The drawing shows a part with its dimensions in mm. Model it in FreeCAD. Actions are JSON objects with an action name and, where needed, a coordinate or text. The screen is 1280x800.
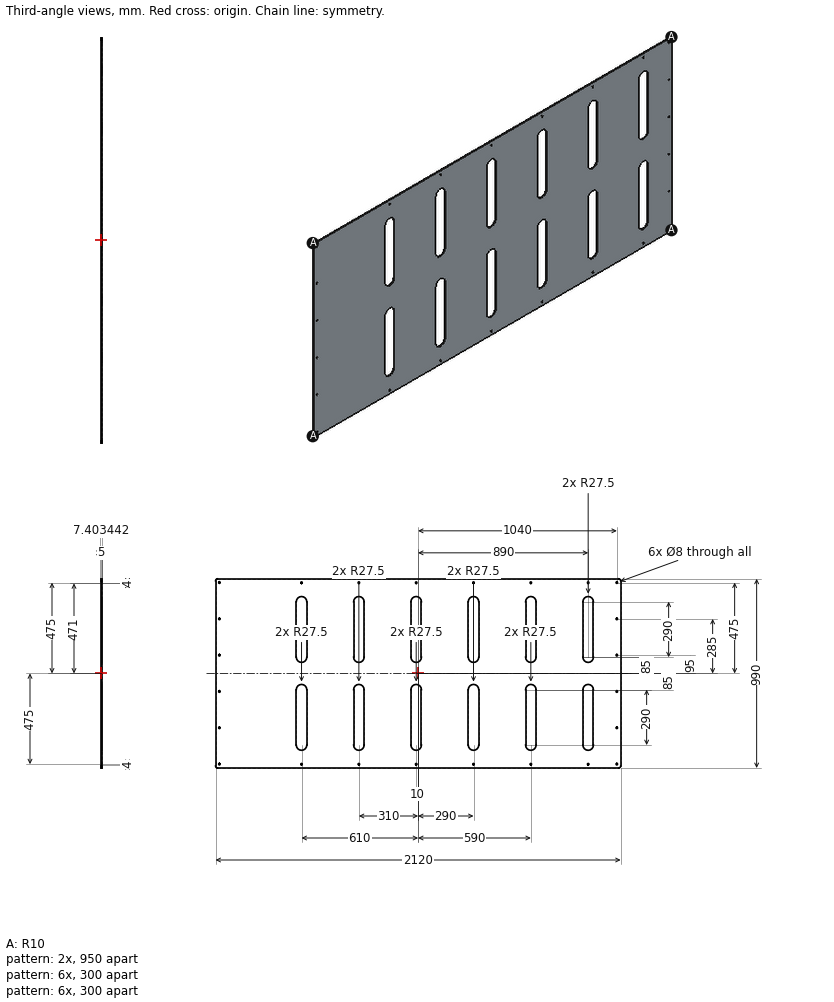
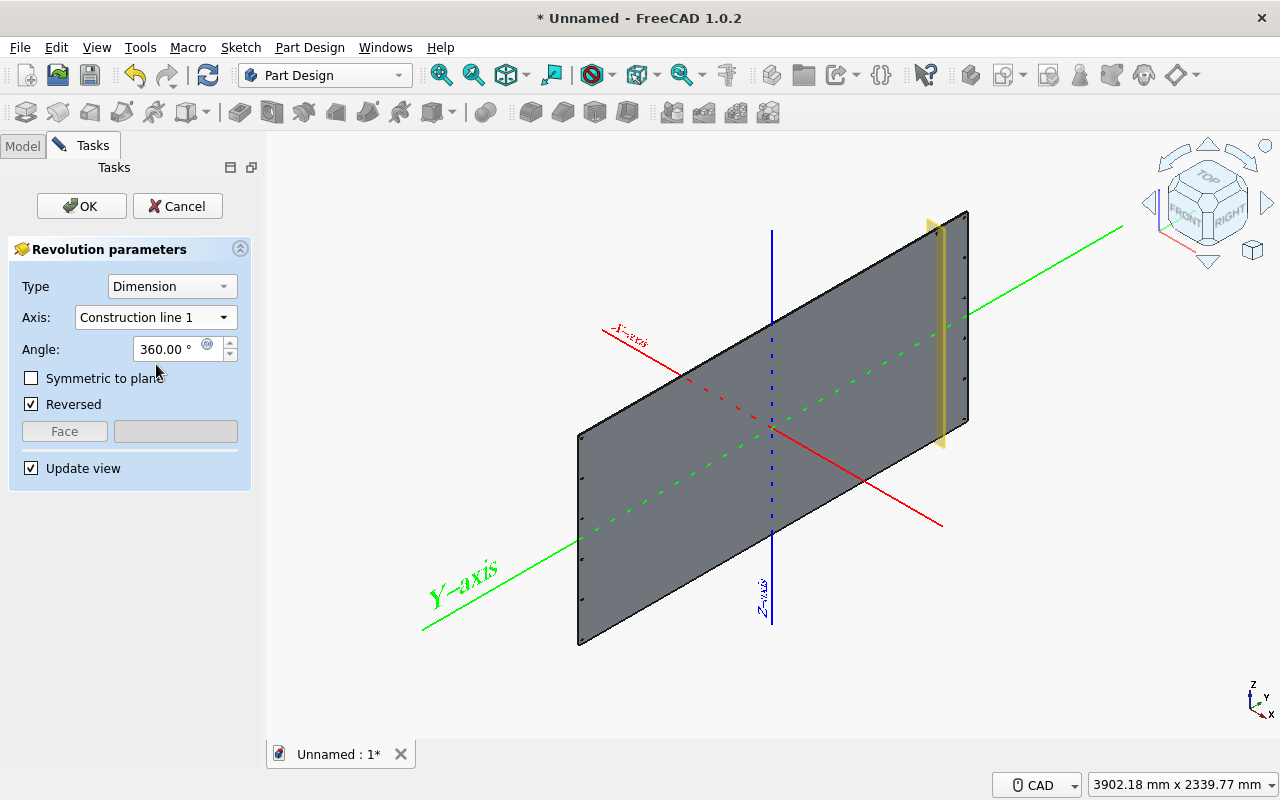
{"action": "left_click", "coordinate": [82, 206]}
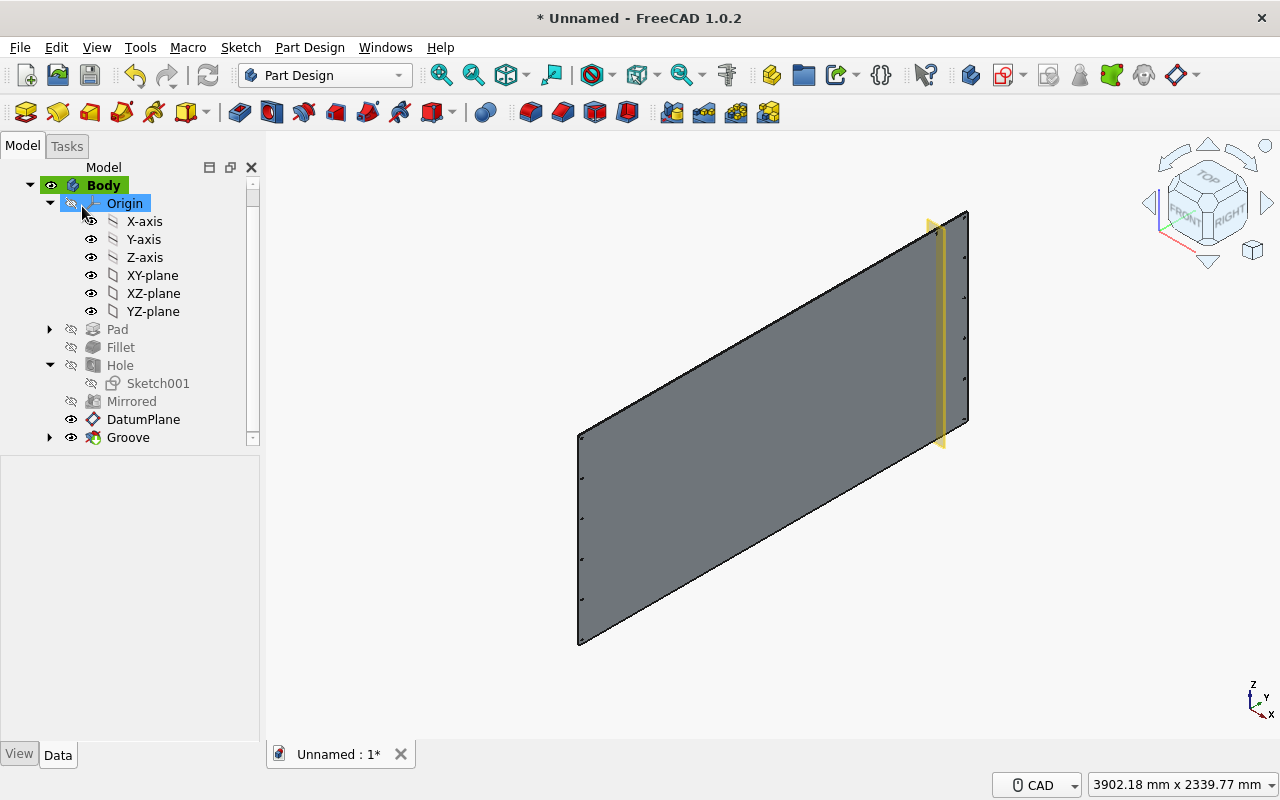
{"action": "left_click", "coordinate": [116, 419]}
{"action": "key", "text": "space"}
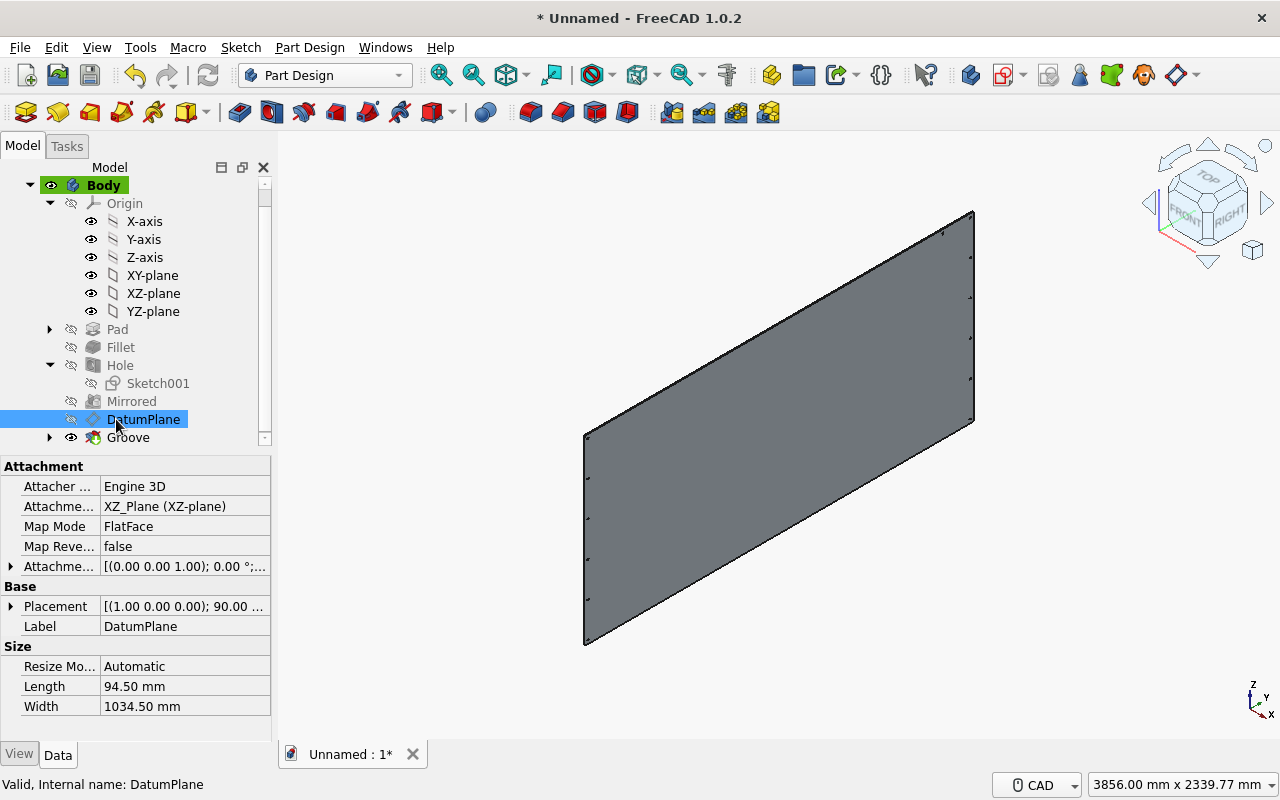
{"action": "left_click", "coordinate": [116, 437]}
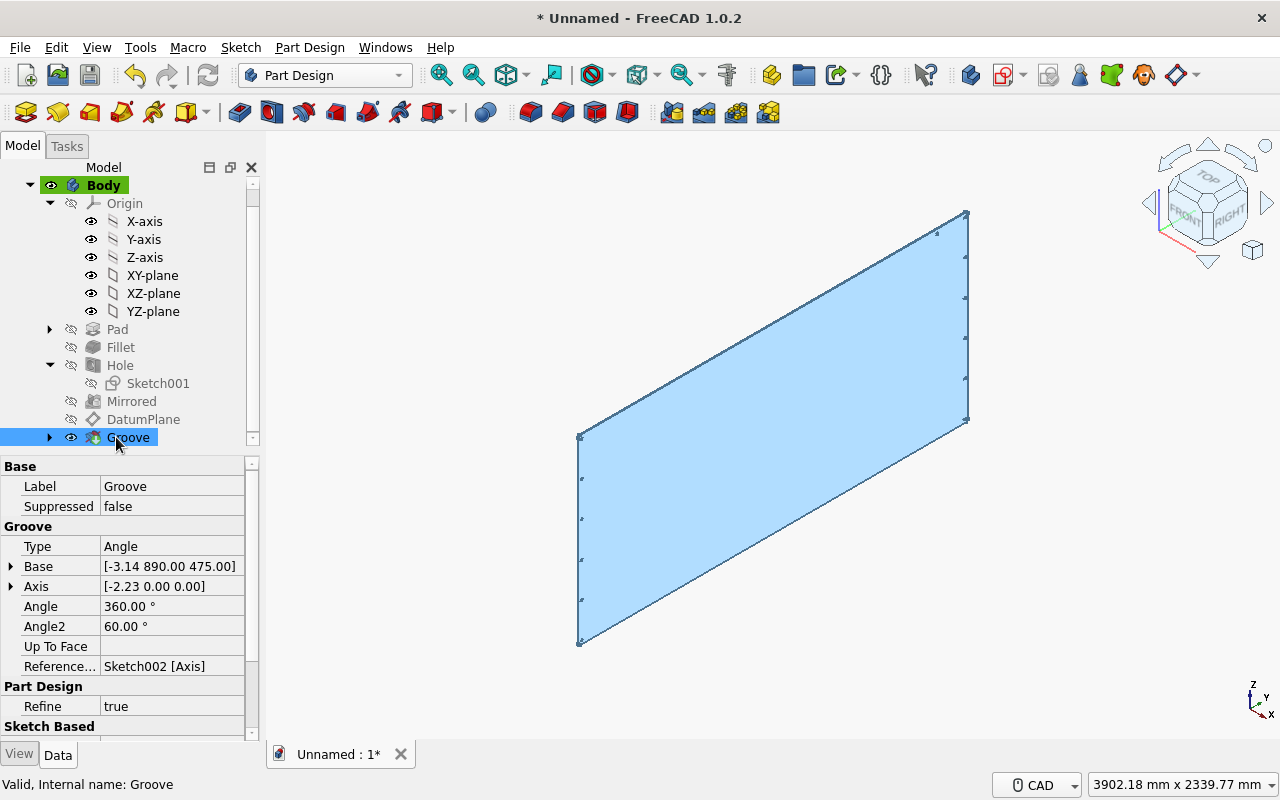
{"action": "left_click", "coordinate": [704, 112]}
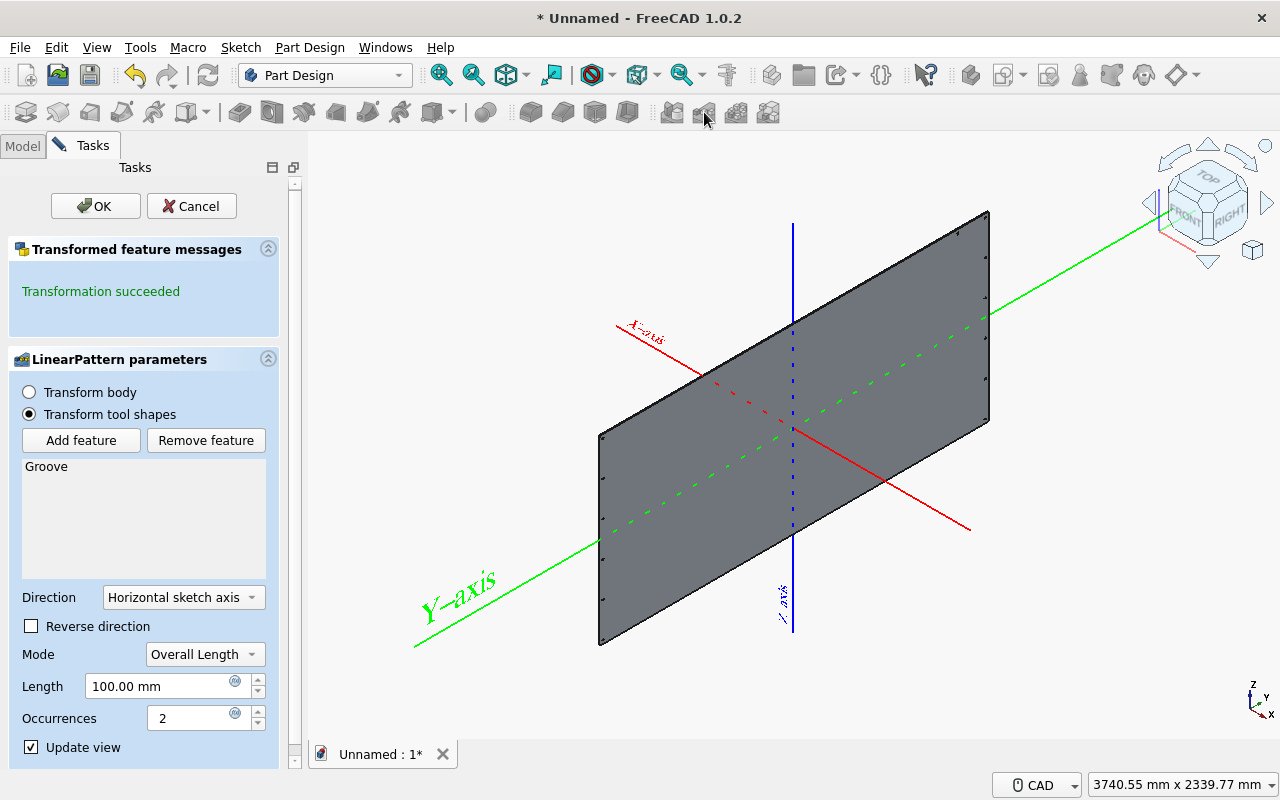
{"action": "left_click", "coordinate": [184, 598]}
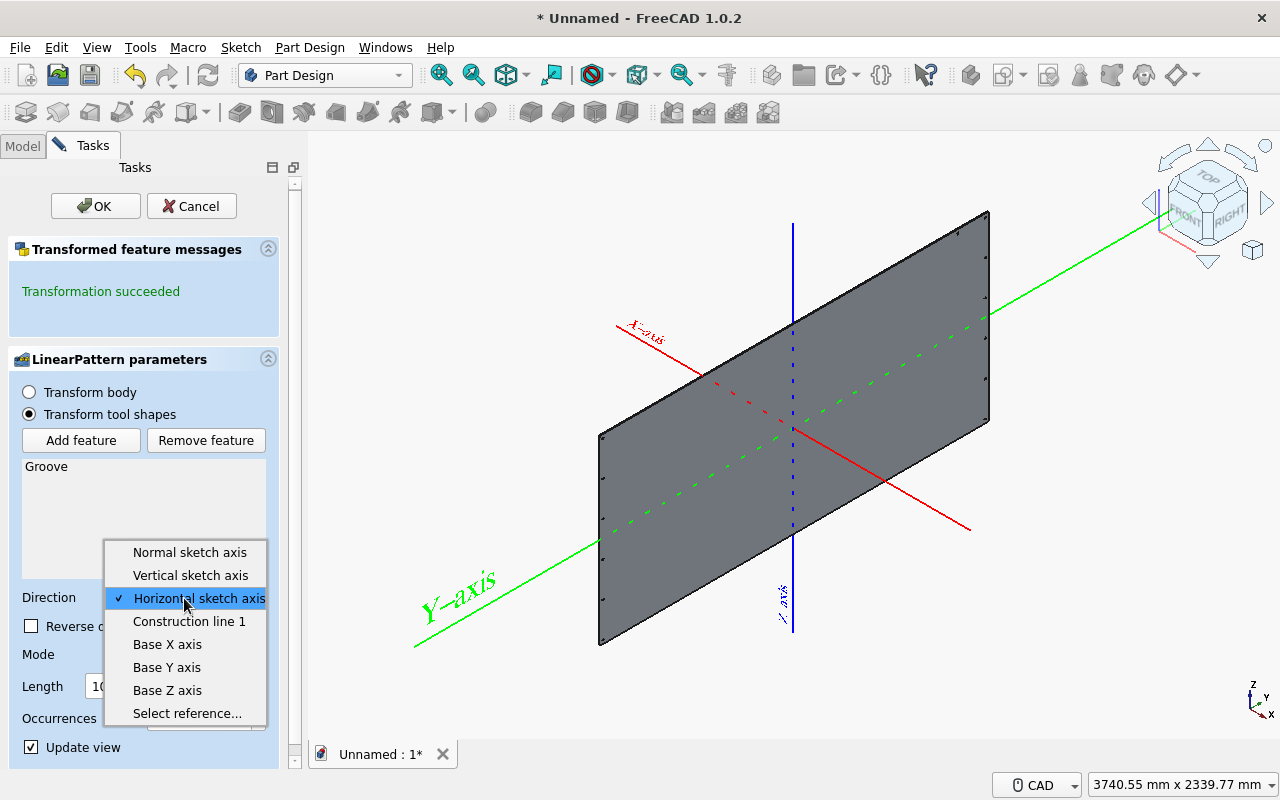
{"action": "left_click", "coordinate": [184, 690]}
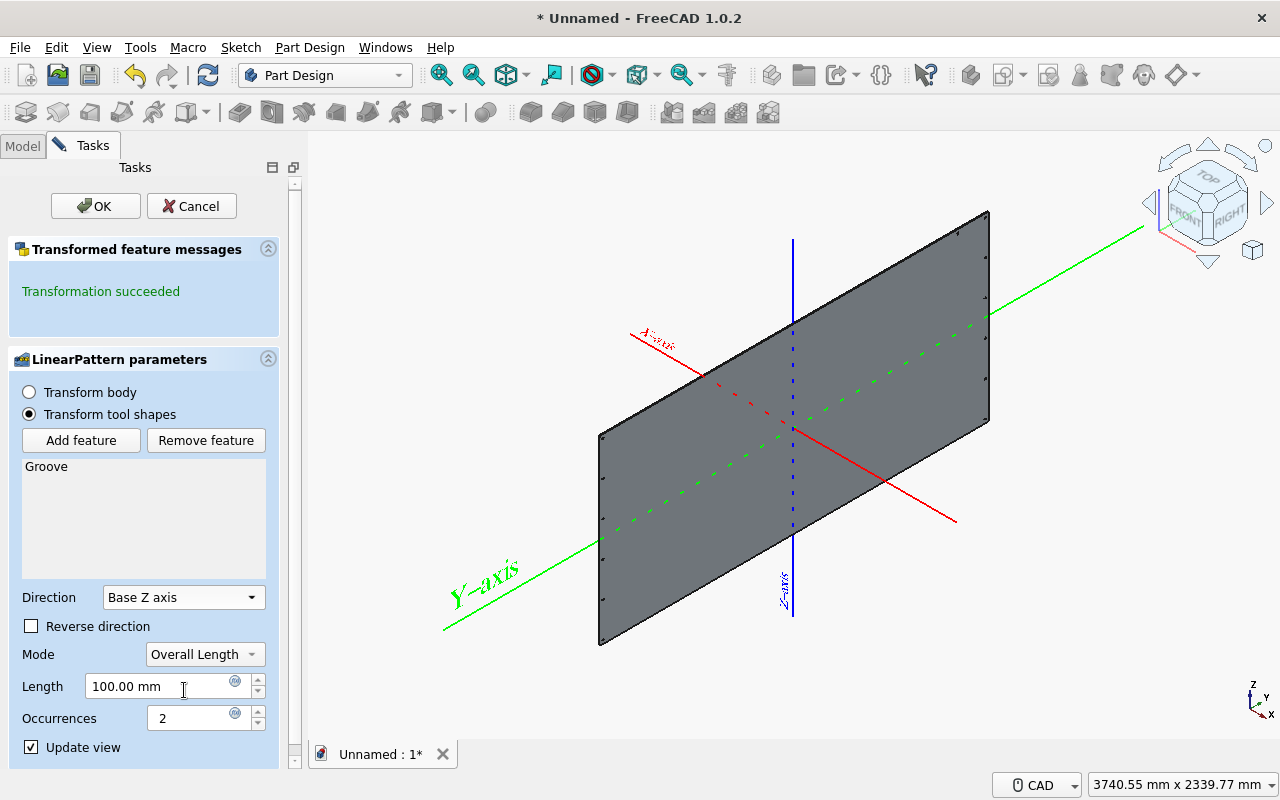
{"action": "left_click", "coordinate": [206, 654]}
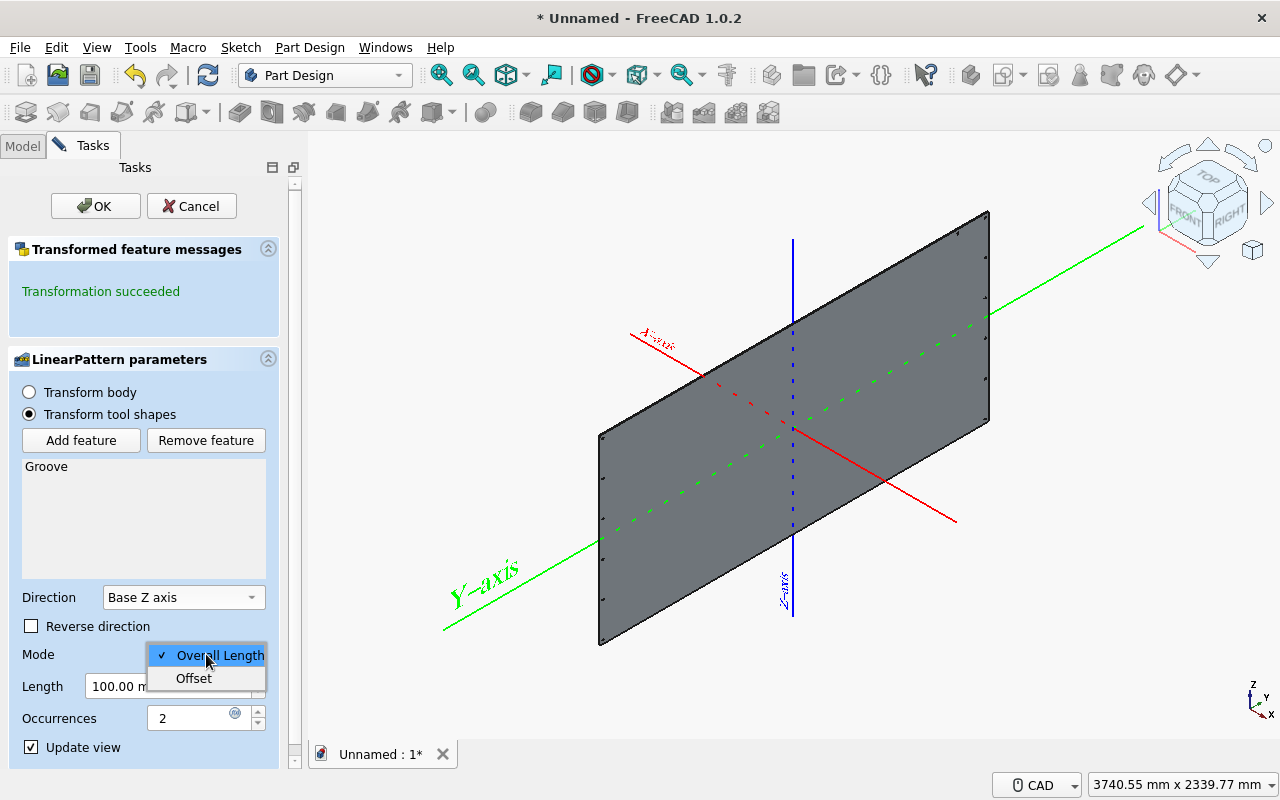
{"action": "left_click", "coordinate": [206, 678]}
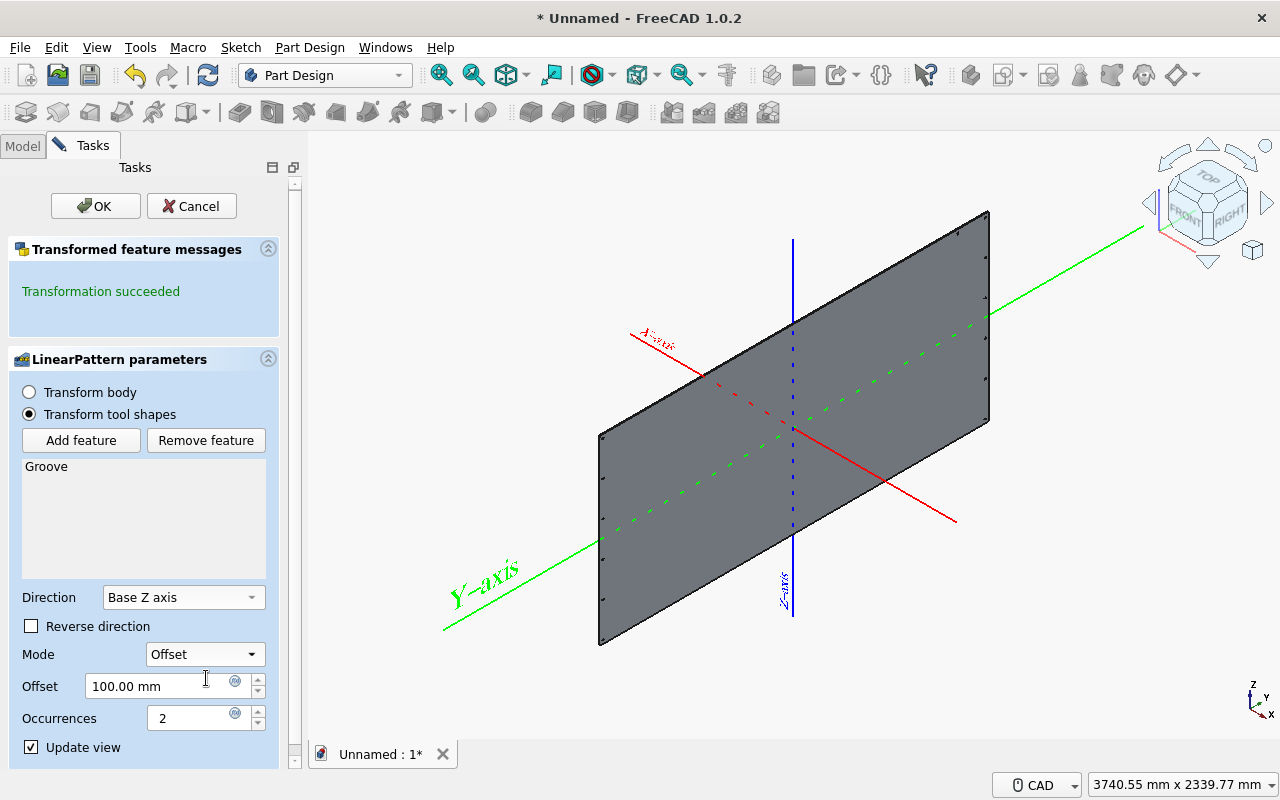
{"action": "triple_click", "coordinate": [168, 686]}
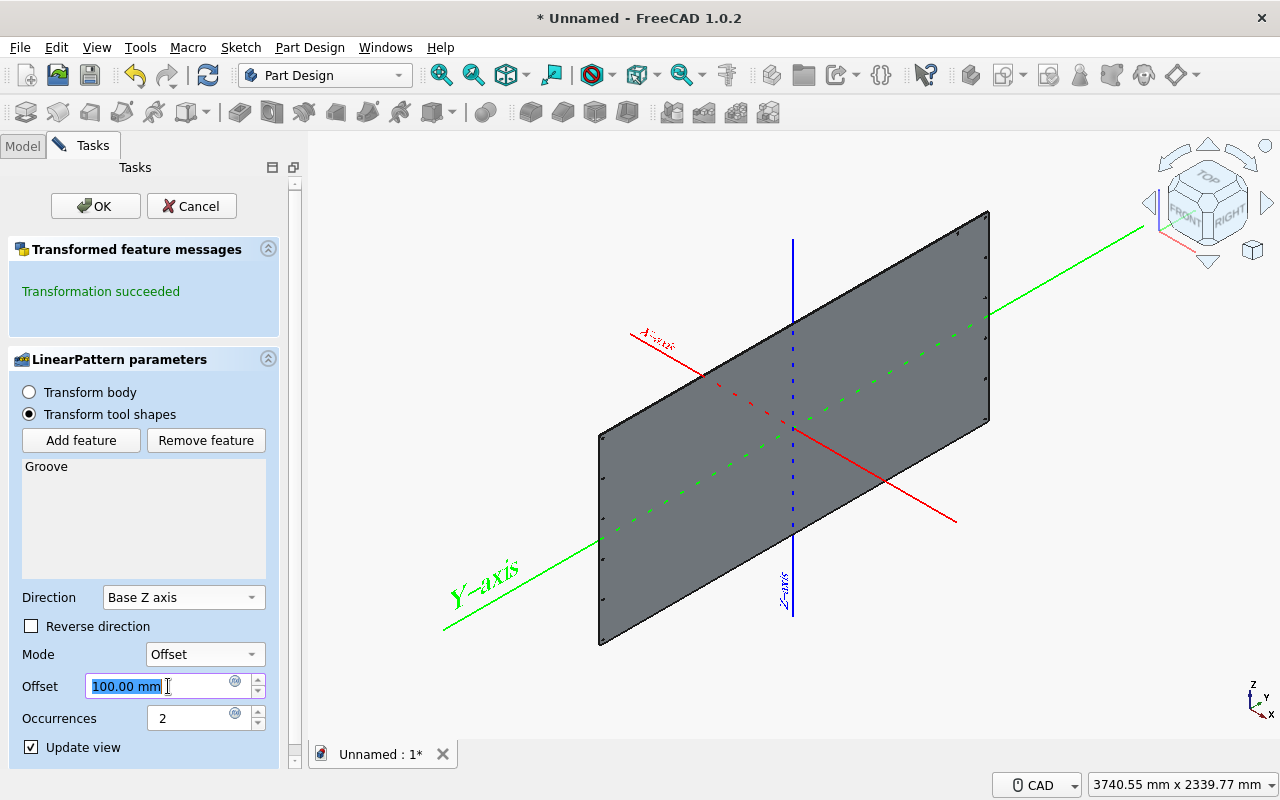
{"action": "type", "text": "950"}
{"action": "key", "text": "Tab"}